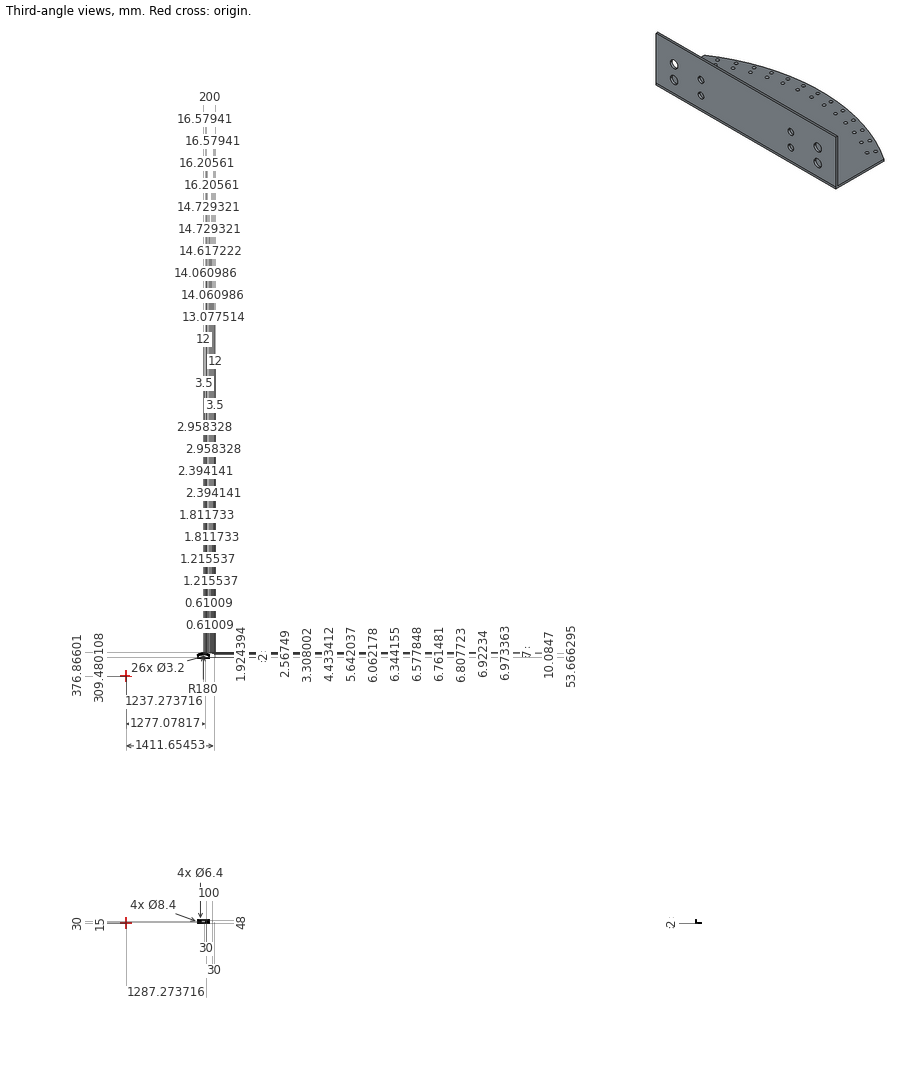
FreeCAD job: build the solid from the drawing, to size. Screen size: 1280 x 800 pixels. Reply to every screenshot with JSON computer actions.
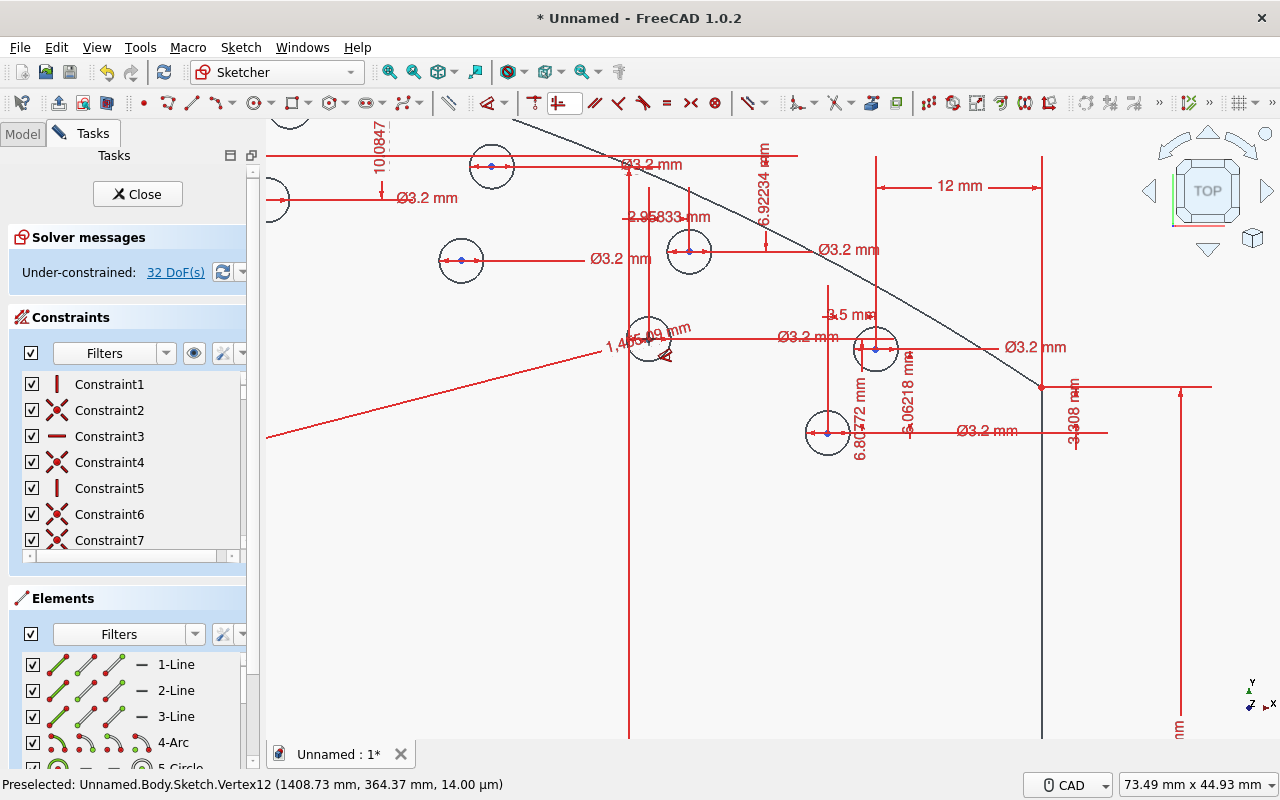
{"action": "left_click", "coordinate": [689, 252]}
{"action": "left_click", "coordinate": [723, 295]}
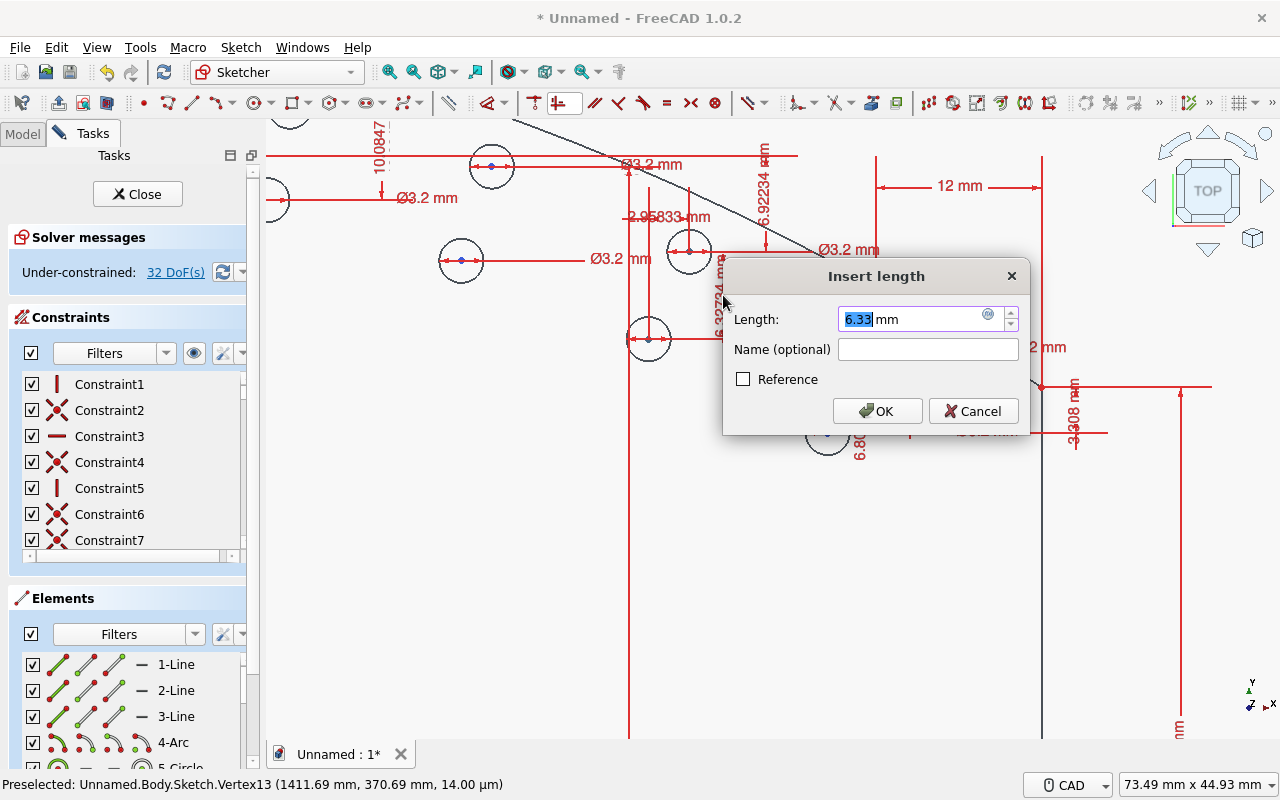
{"action": "type", "text": "6.344155"}
{"action": "key", "text": "Return"}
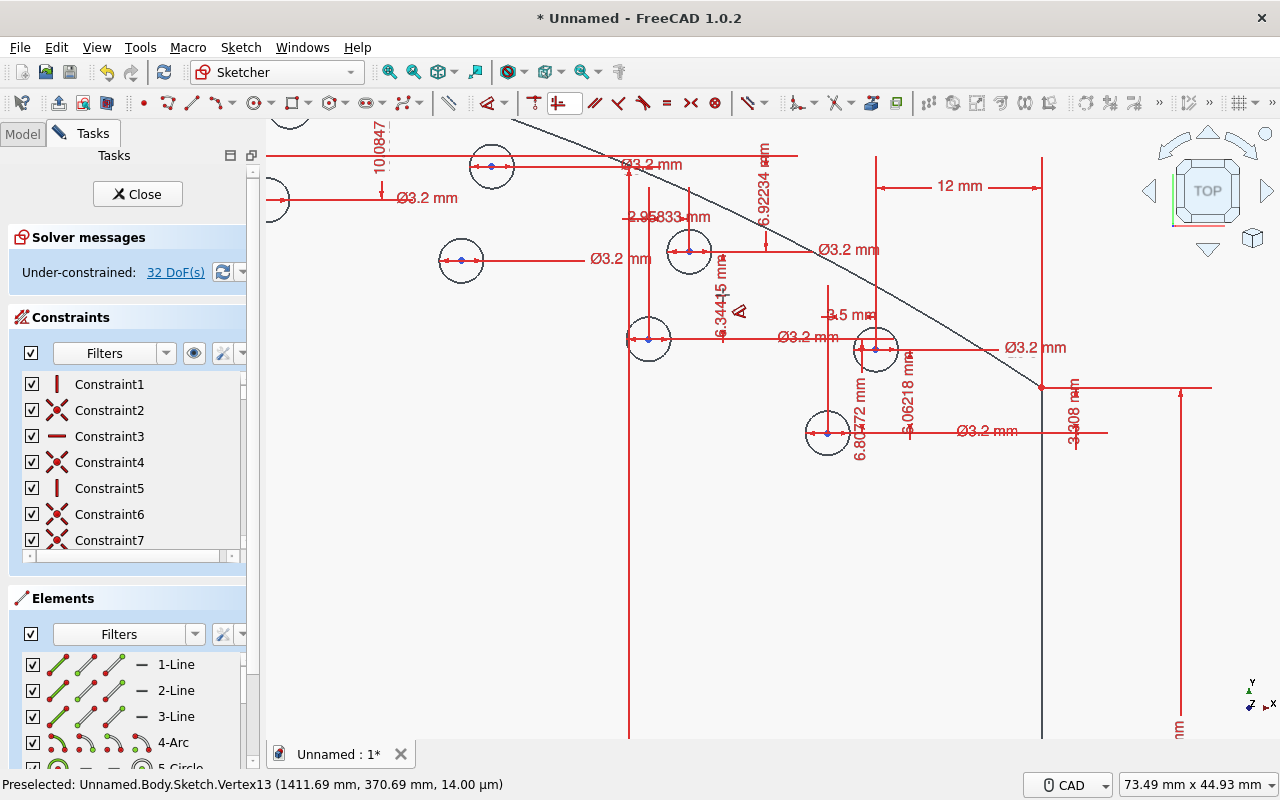
{"action": "scroll", "coordinate": [968, 400], "scroll_direction": "down", "scroll_amount": 8}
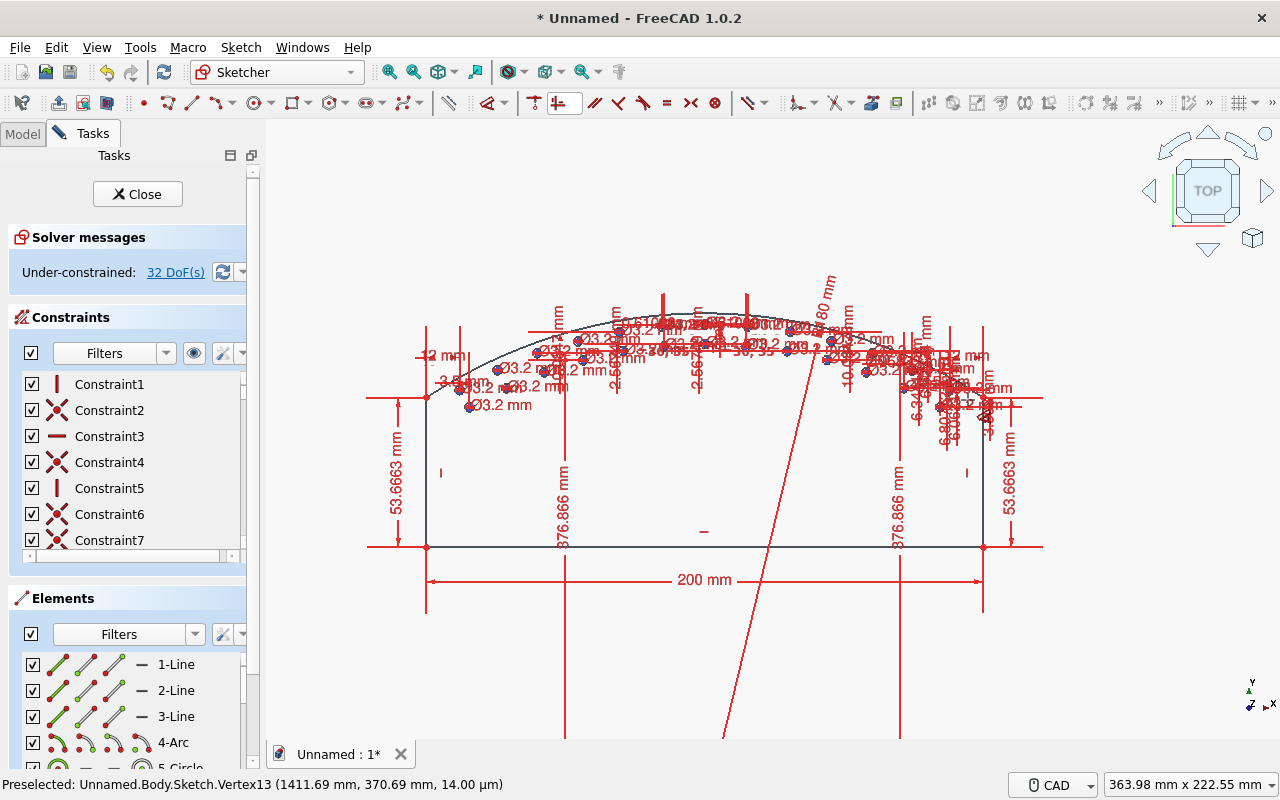
{"action": "left_click", "coordinate": [912, 370]}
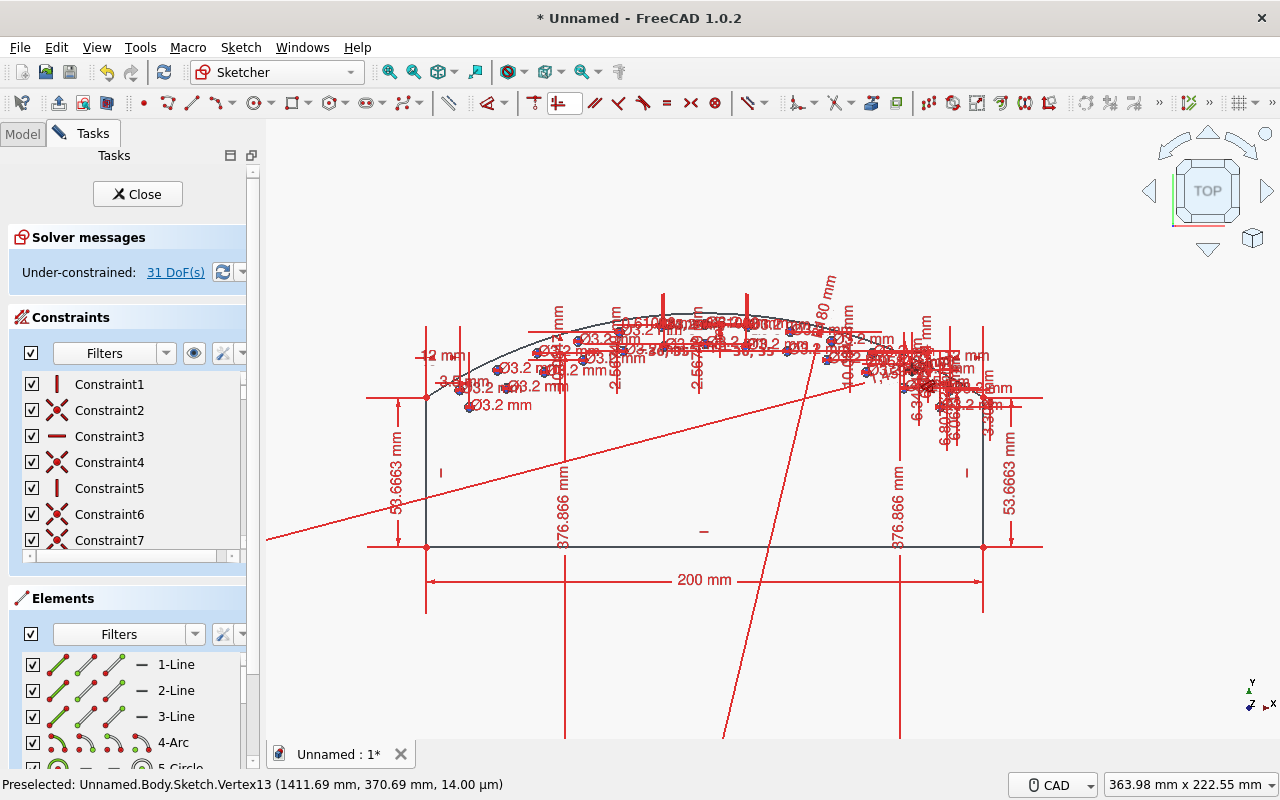
{"action": "left_click", "coordinate": [866, 372]}
{"action": "left_click", "coordinate": [873, 406]}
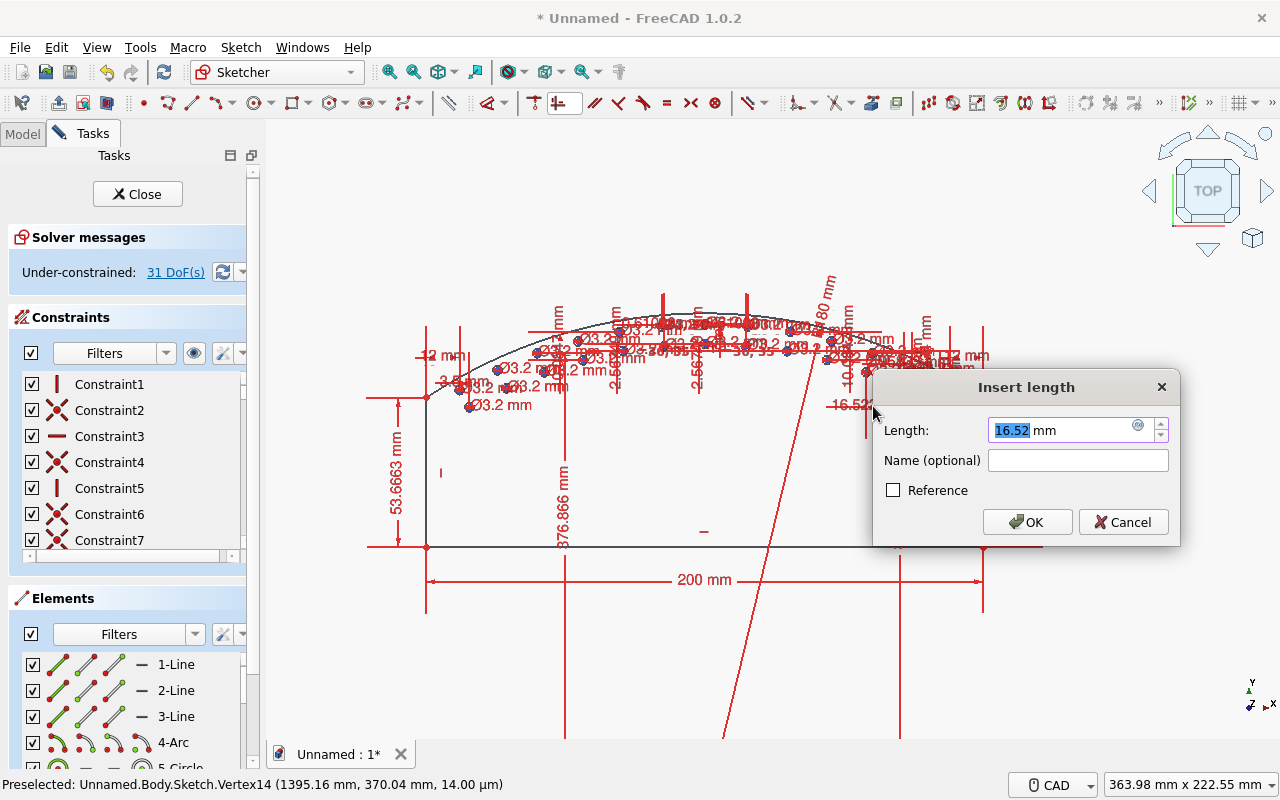
{"action": "type", "text": "16.57941"}
{"action": "key", "text": "Return"}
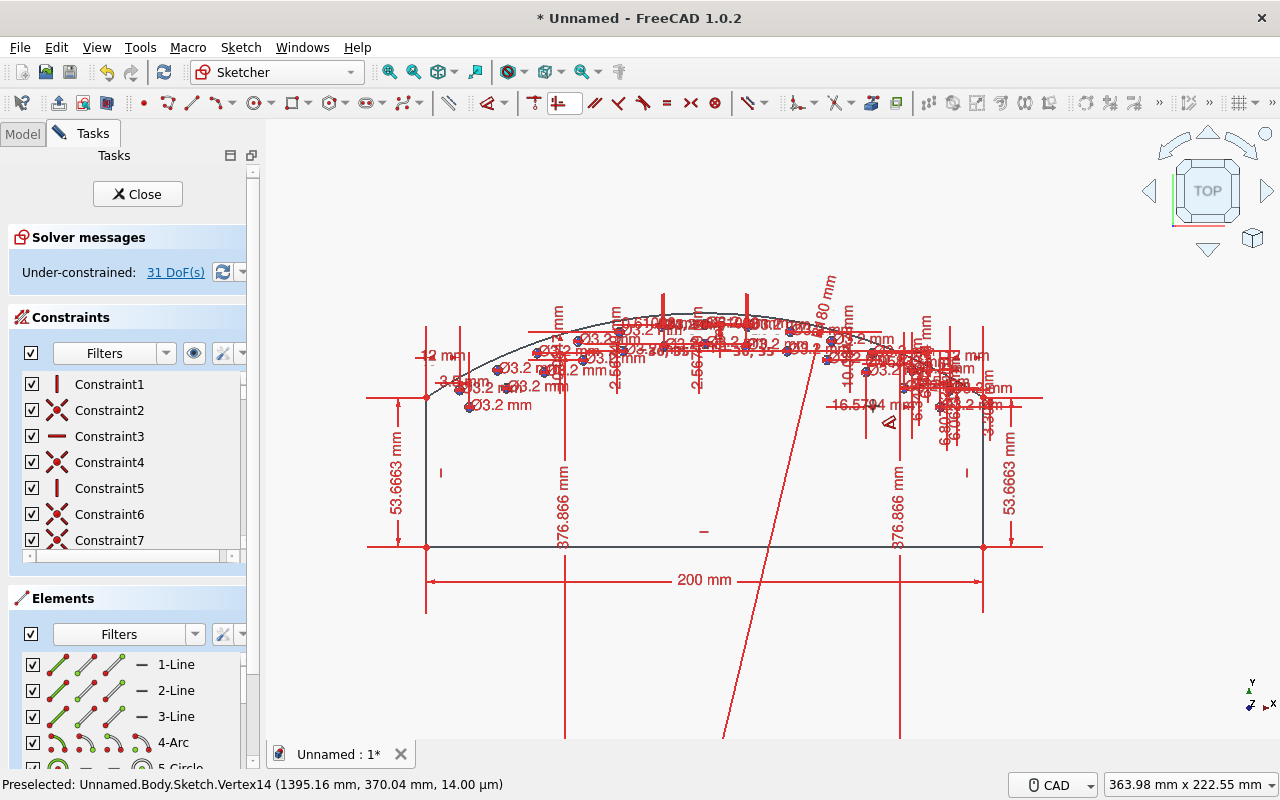
{"action": "scroll", "coordinate": [904, 388], "scroll_direction": "up", "scroll_amount": 5}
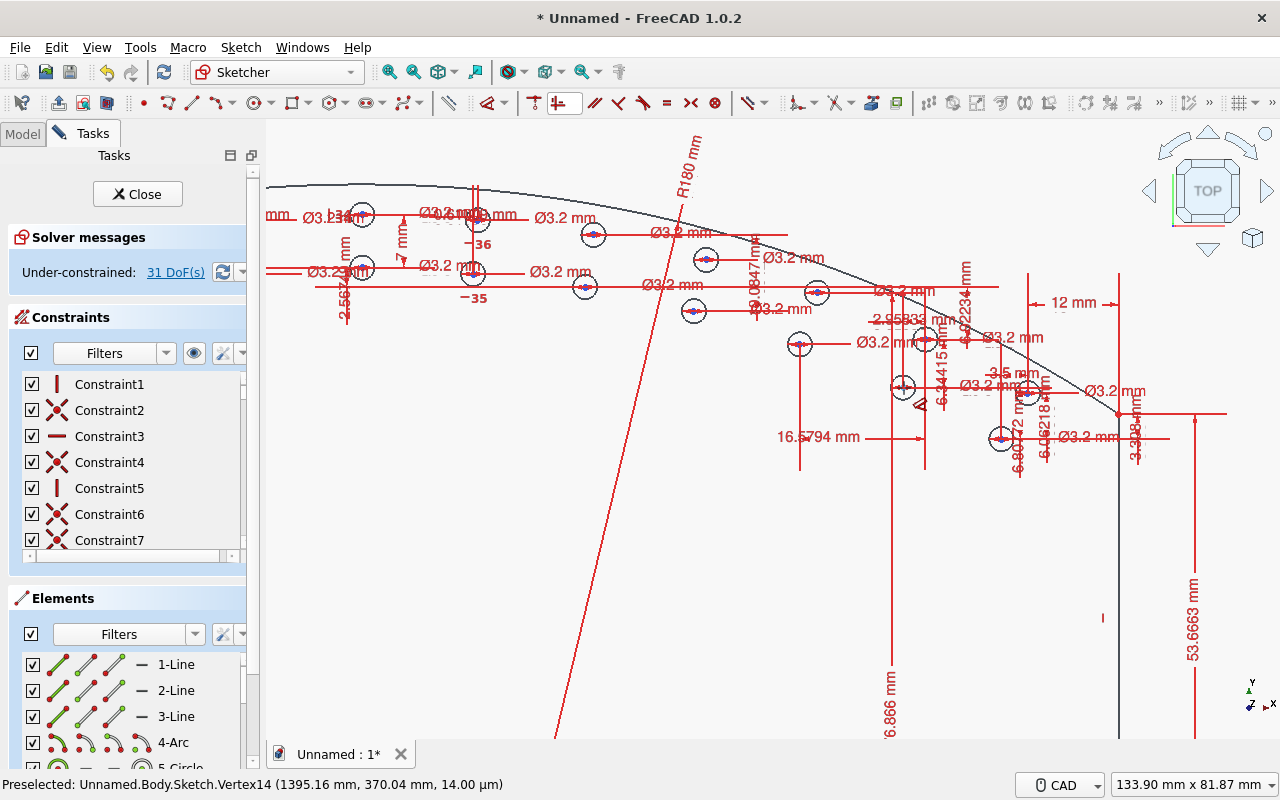
{"action": "left_click", "coordinate": [903, 388]}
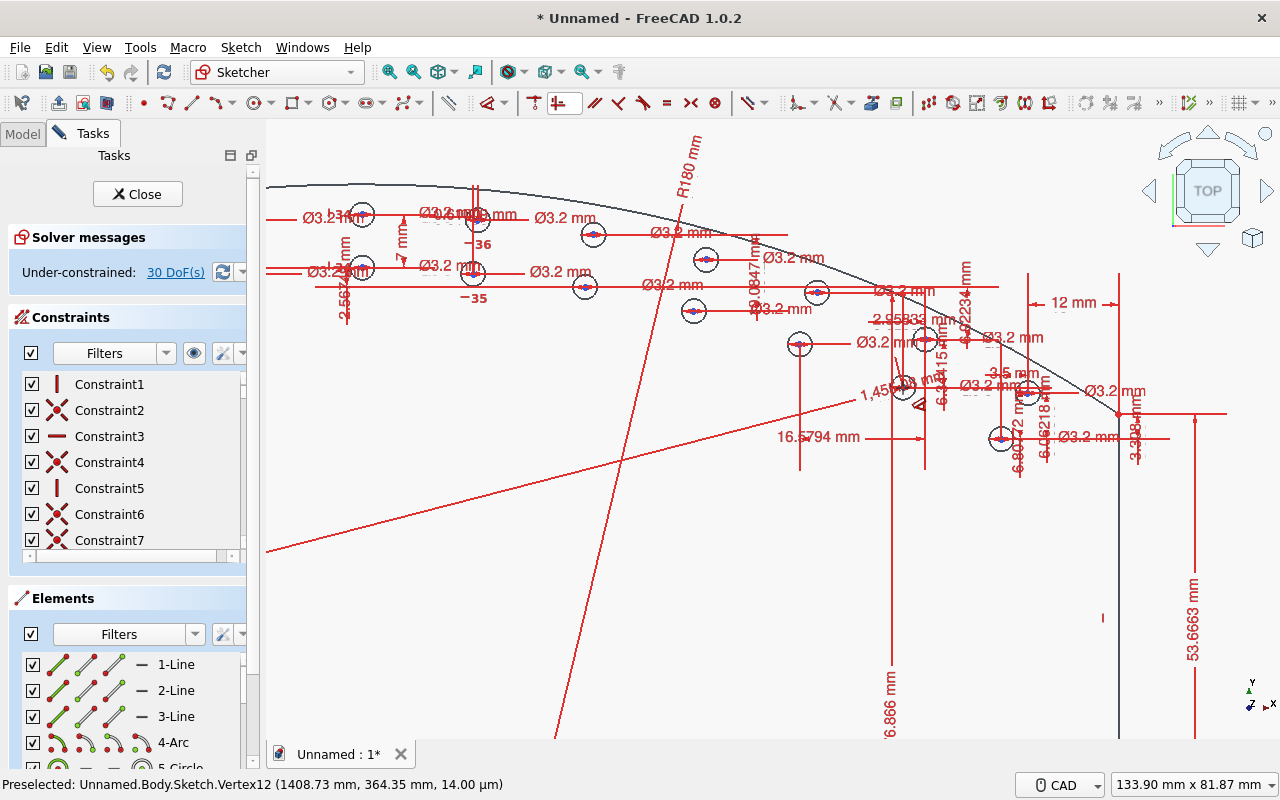
{"action": "left_click", "coordinate": [800, 344]}
{"action": "left_click", "coordinate": [766, 366]}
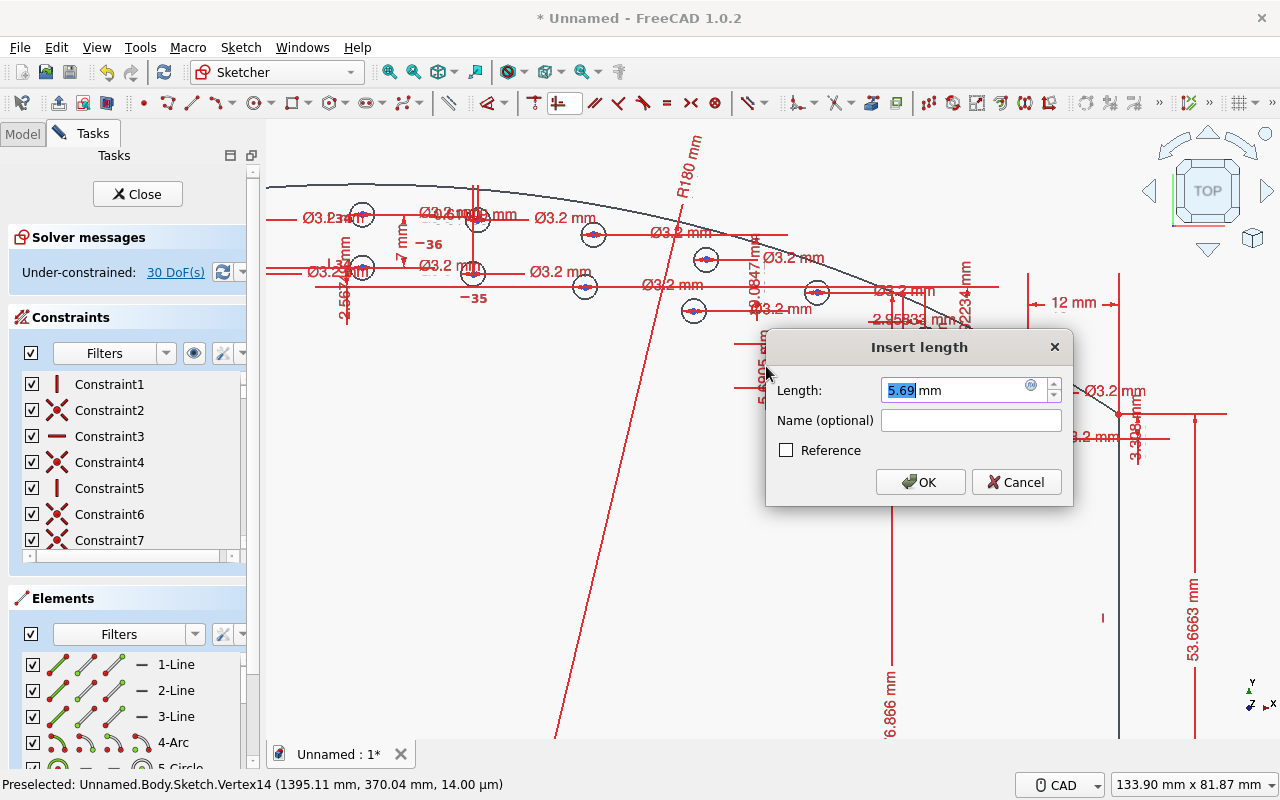
{"action": "type", "text": "5.642037"}
{"action": "key", "text": "Return"}